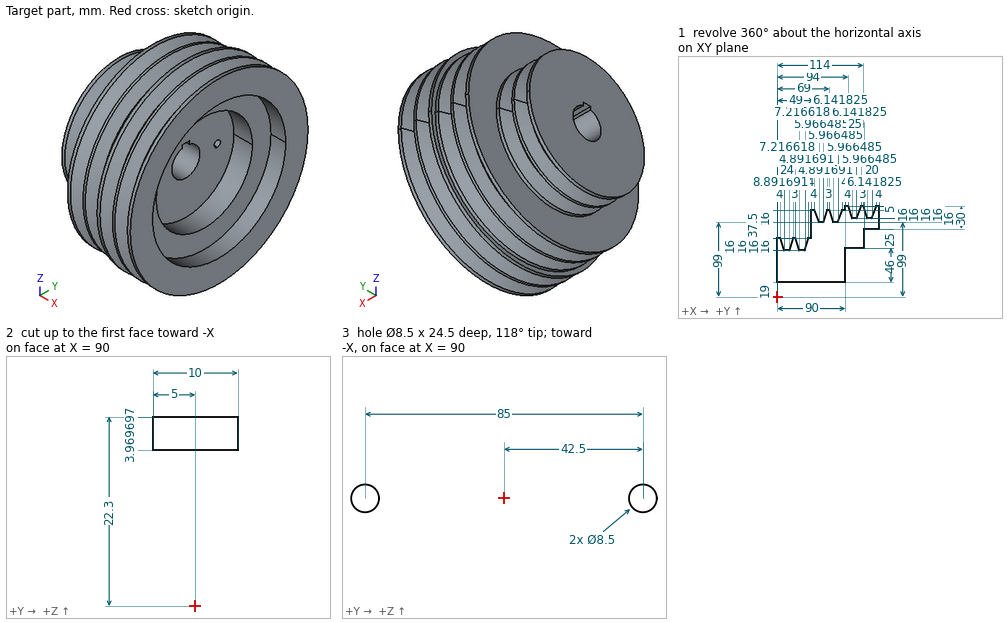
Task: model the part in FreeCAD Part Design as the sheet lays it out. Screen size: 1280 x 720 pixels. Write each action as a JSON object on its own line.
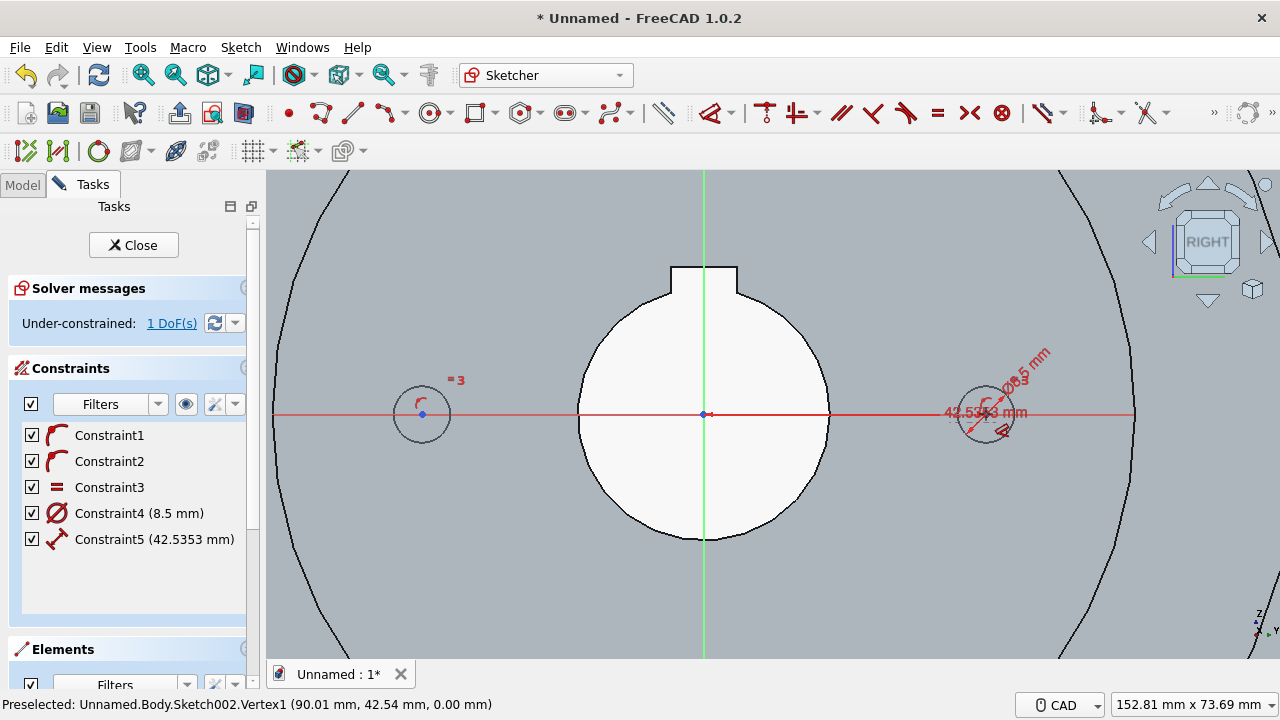
{"action": "left_click", "coordinate": [422, 414]}
{"action": "left_click", "coordinate": [574, 448]}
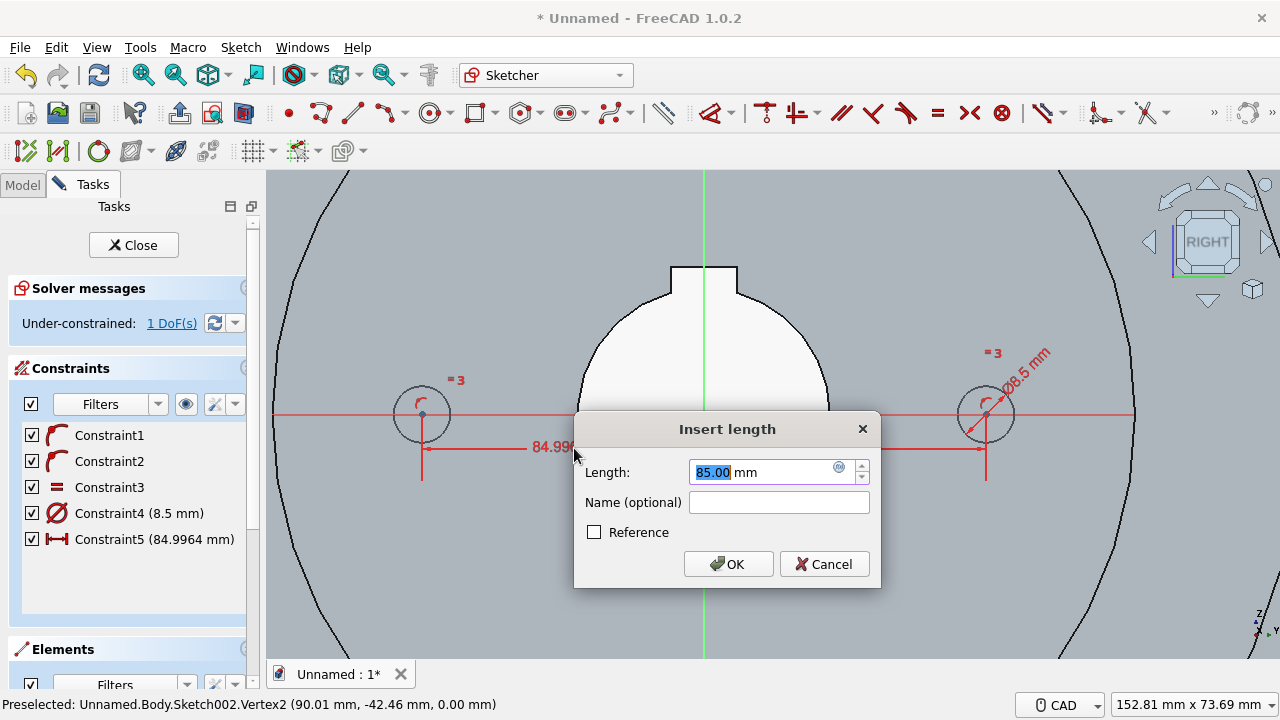
{"action": "type", "text": "85"}
{"action": "key", "text": "Return"}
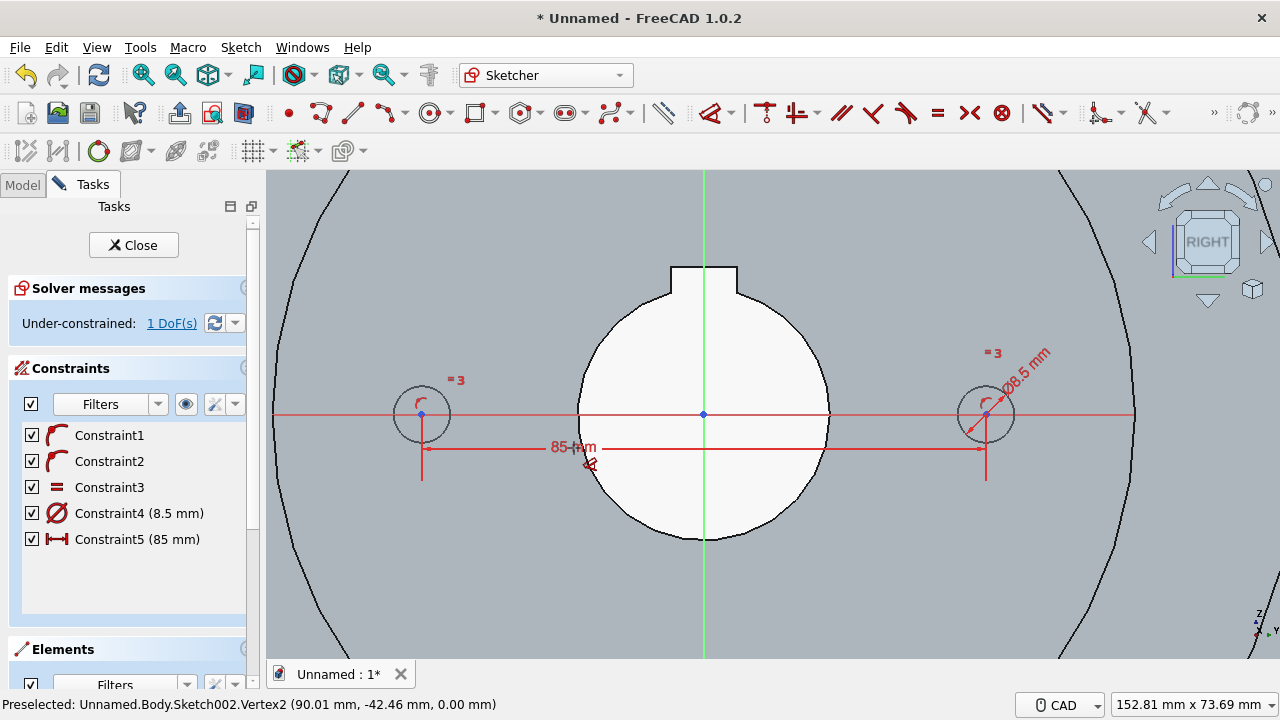
{"action": "left_click", "coordinate": [986, 414]}
{"action": "left_click", "coordinate": [845, 448]}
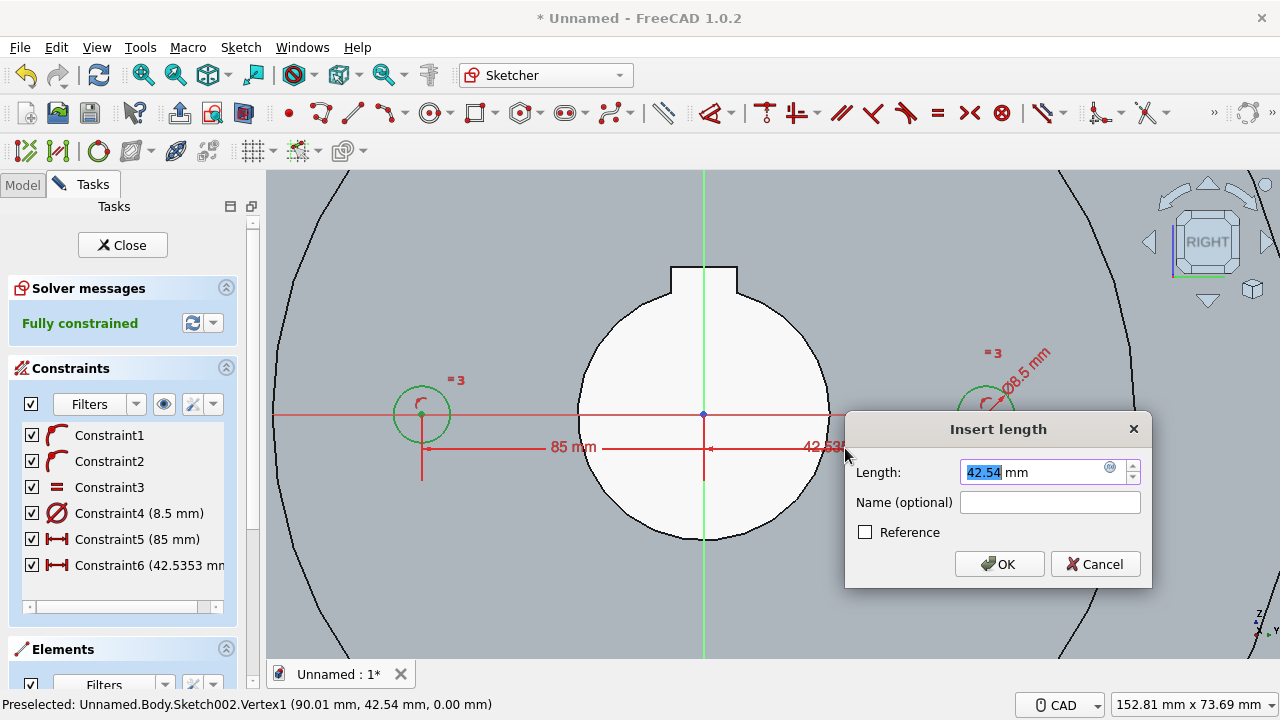
{"action": "type", "text": "42.5"}
{"action": "key", "text": "Return"}
{"action": "key", "text": "Escape"}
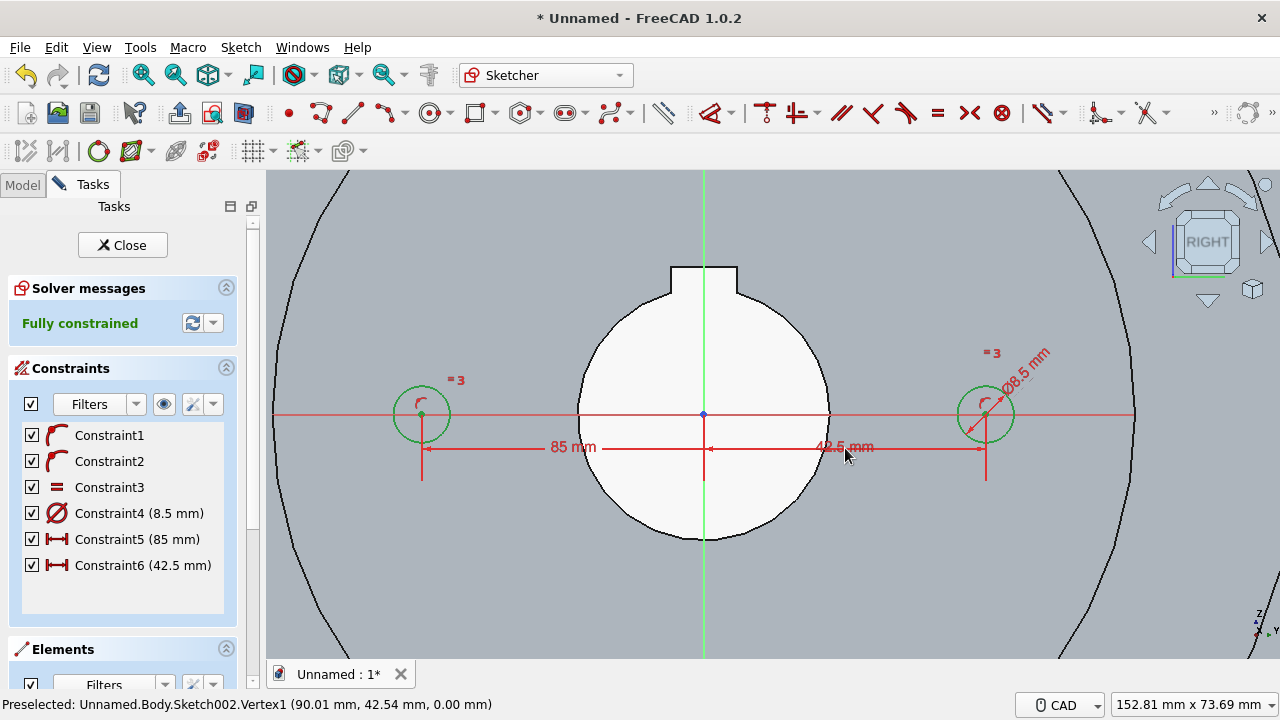
{"action": "left_click", "coordinate": [123, 245]}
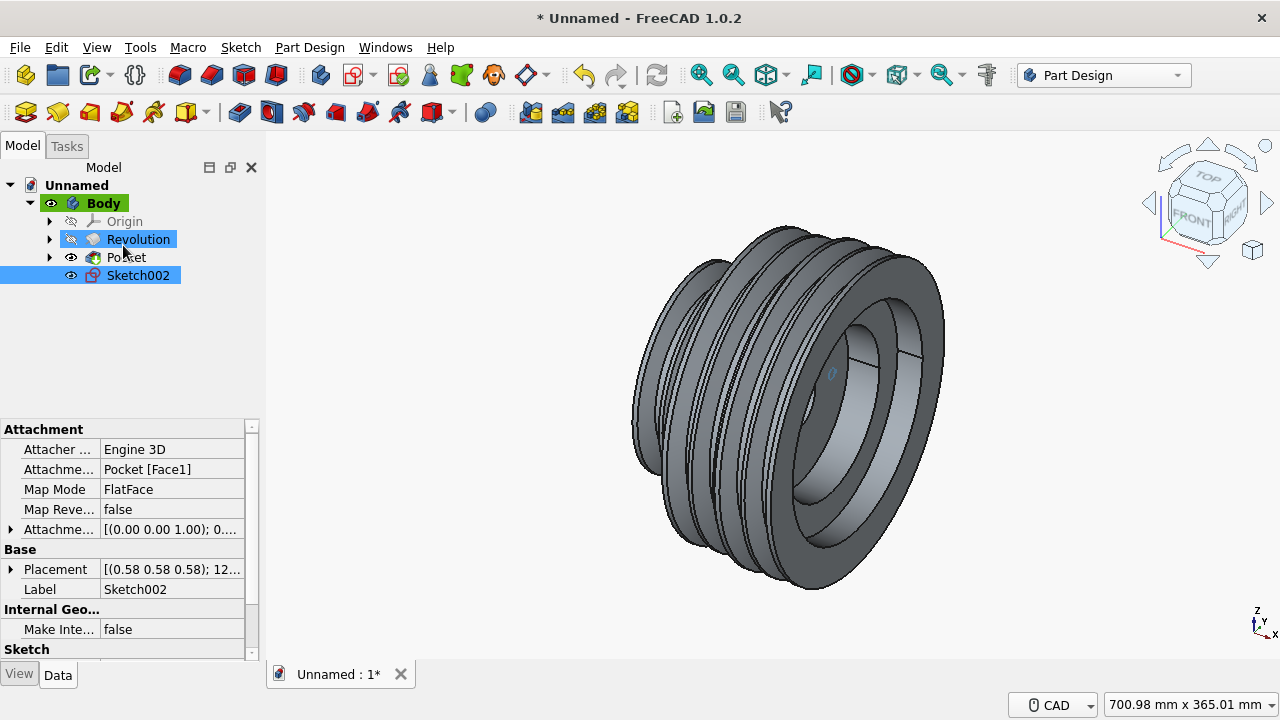
{"action": "left_click", "coordinate": [272, 112]}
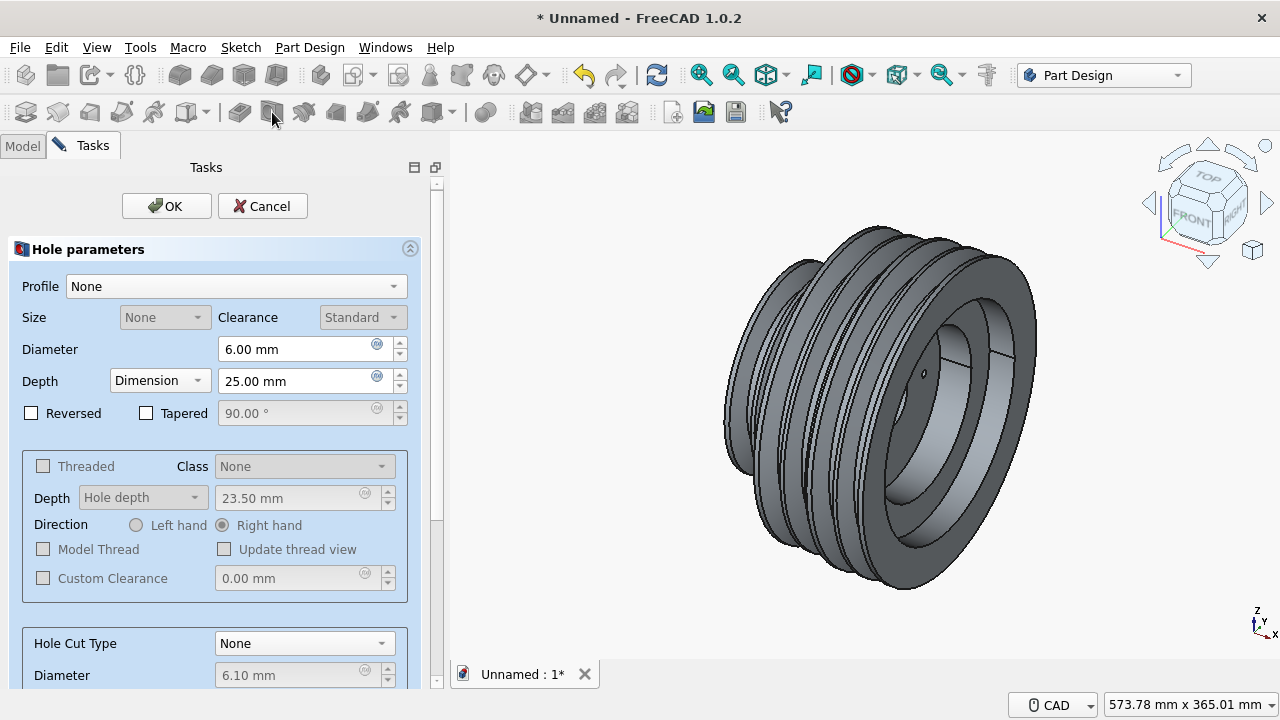
{"action": "triple_click", "coordinate": [305, 349]}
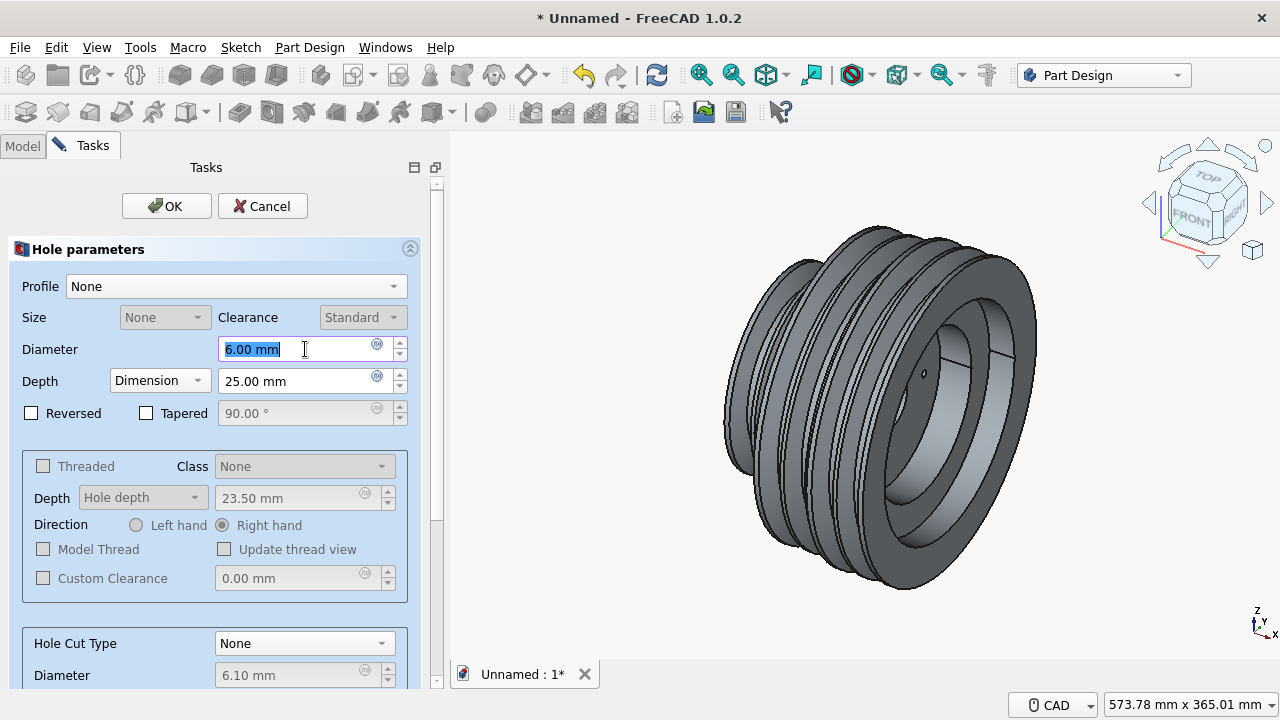
{"action": "type", "text": "8.5"}
{"action": "key", "text": "Tab"}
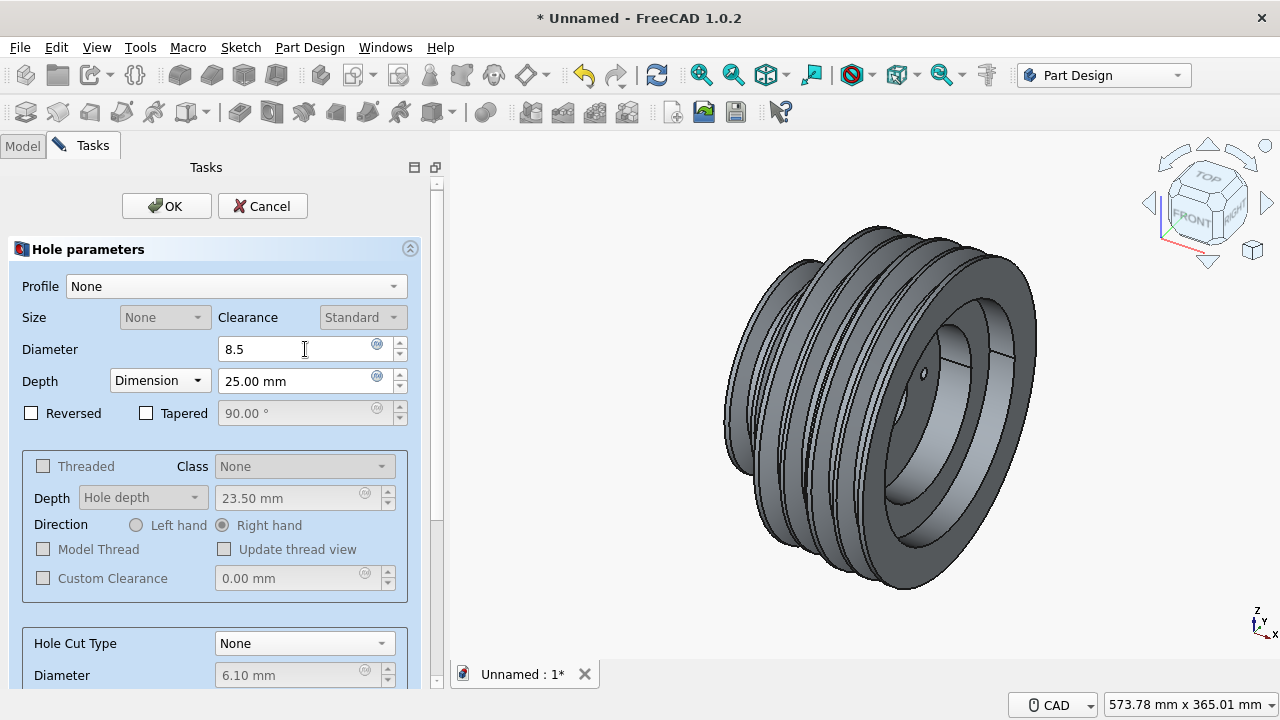
{"action": "triple_click", "coordinate": [305, 381]}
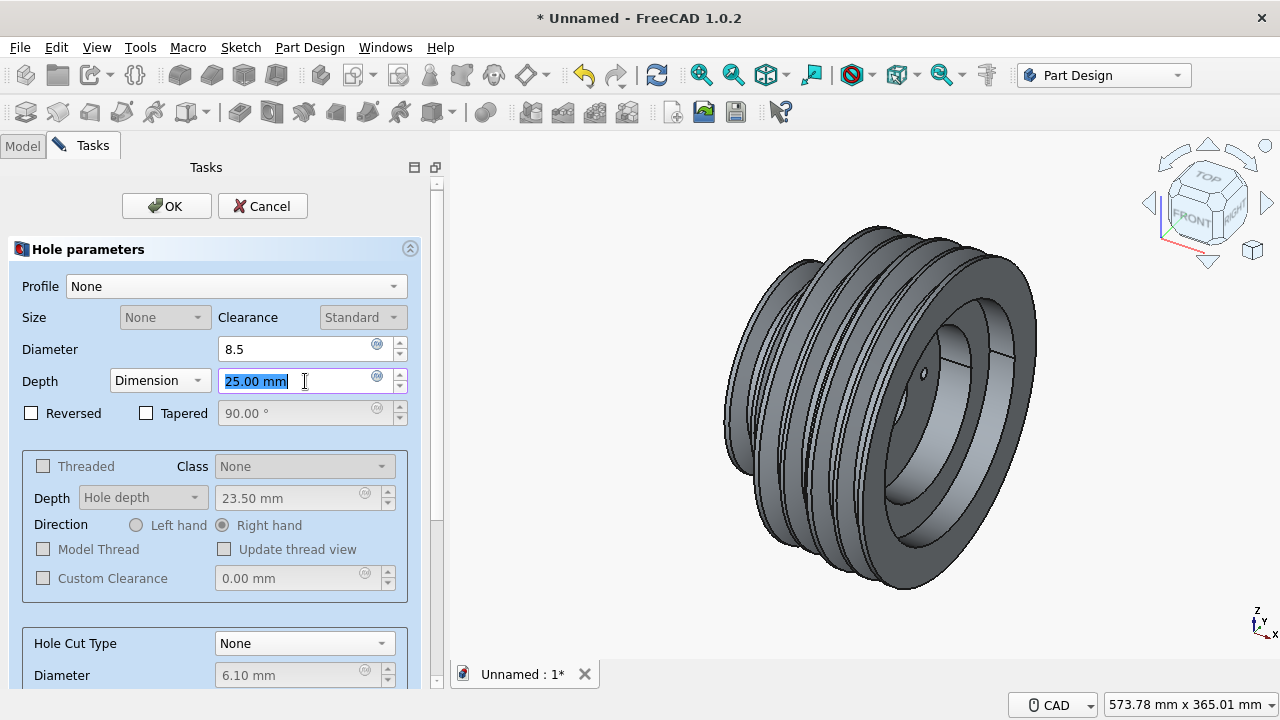
{"action": "type", "text": "24.5"}
{"action": "key", "text": "Tab"}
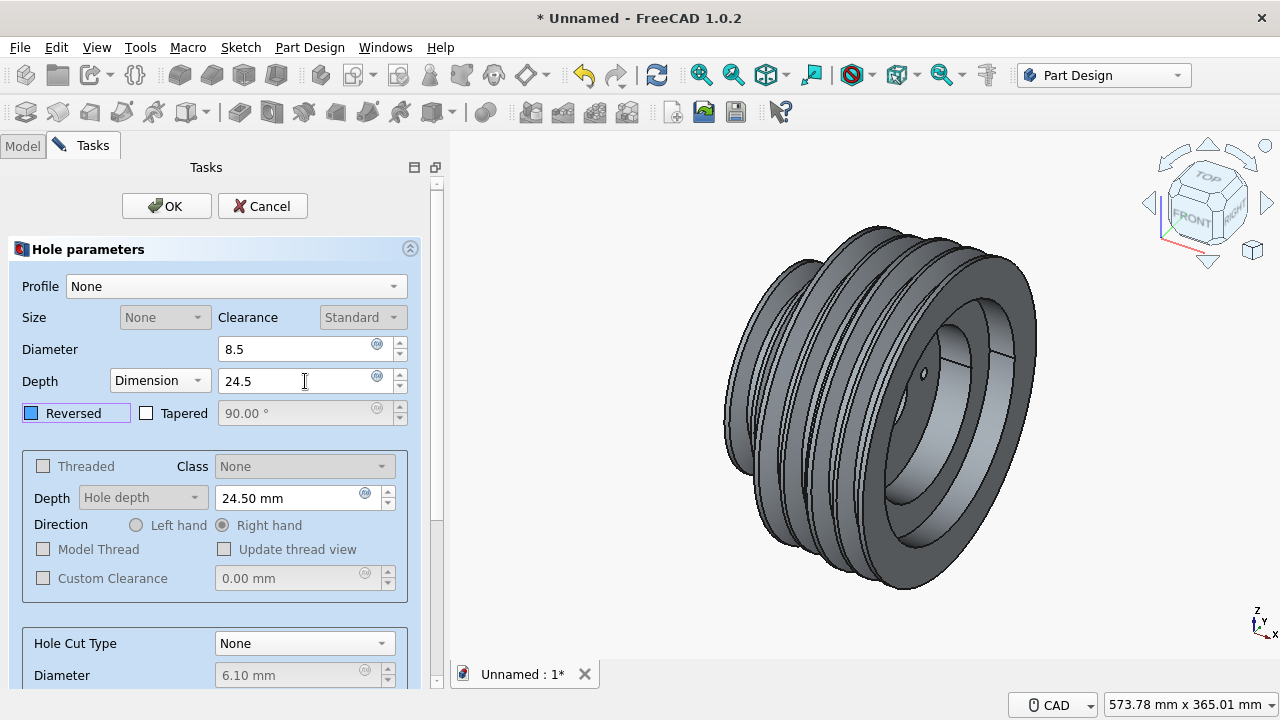
{"action": "left_click", "coordinate": [167, 206]}